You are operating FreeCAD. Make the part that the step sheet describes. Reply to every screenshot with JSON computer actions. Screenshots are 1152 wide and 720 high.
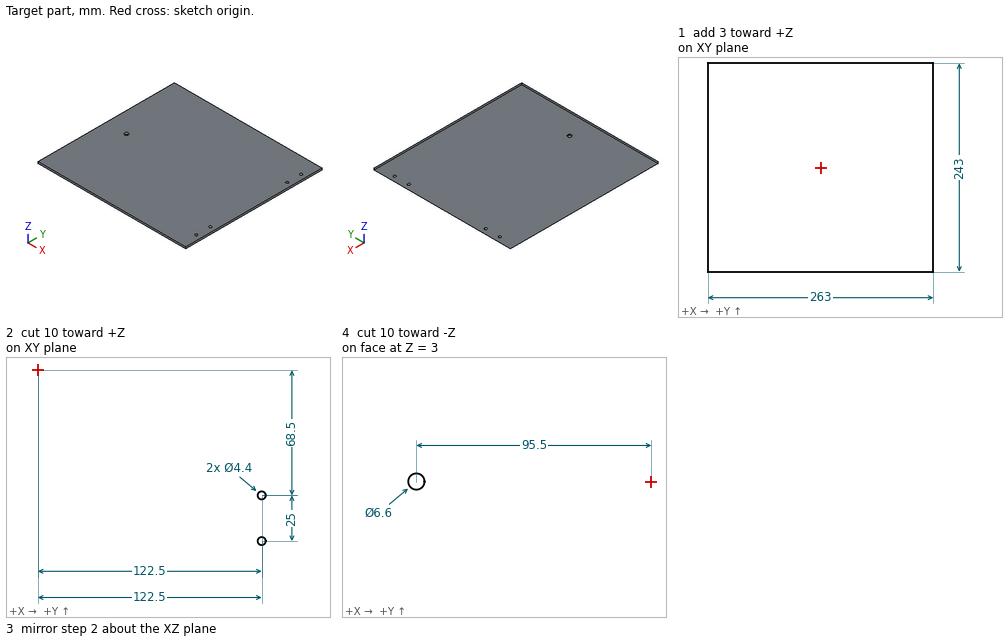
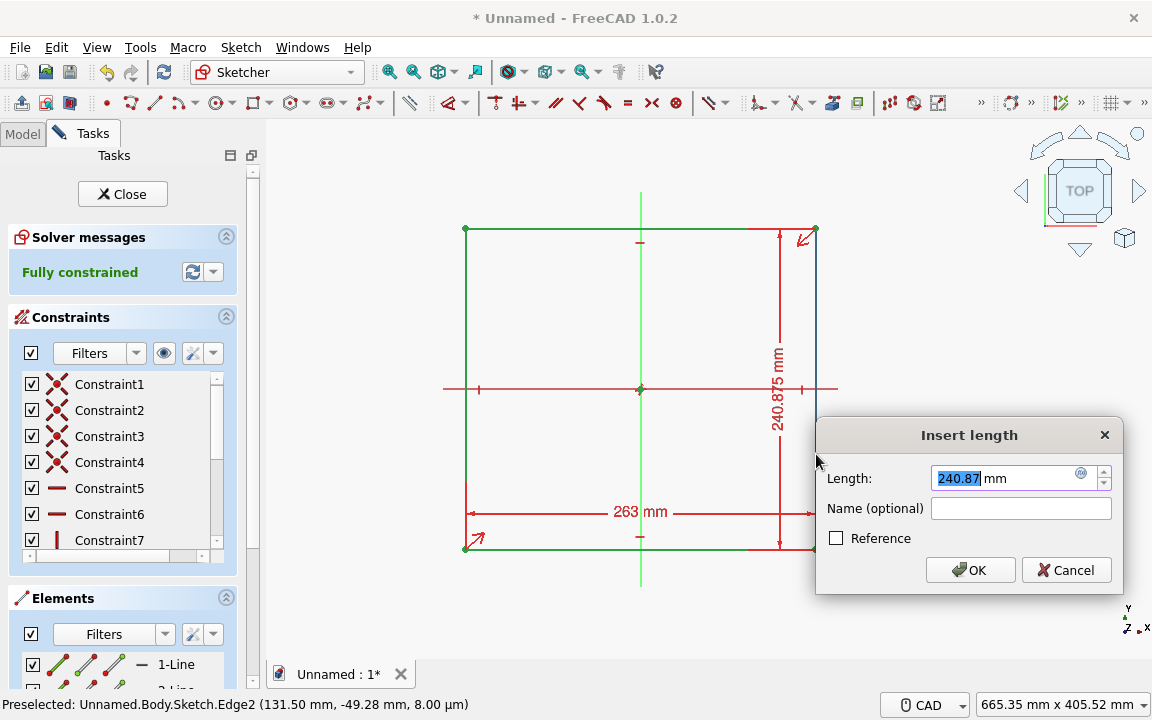
{"action": "type", "text": "243"}
{"action": "key", "text": "Return"}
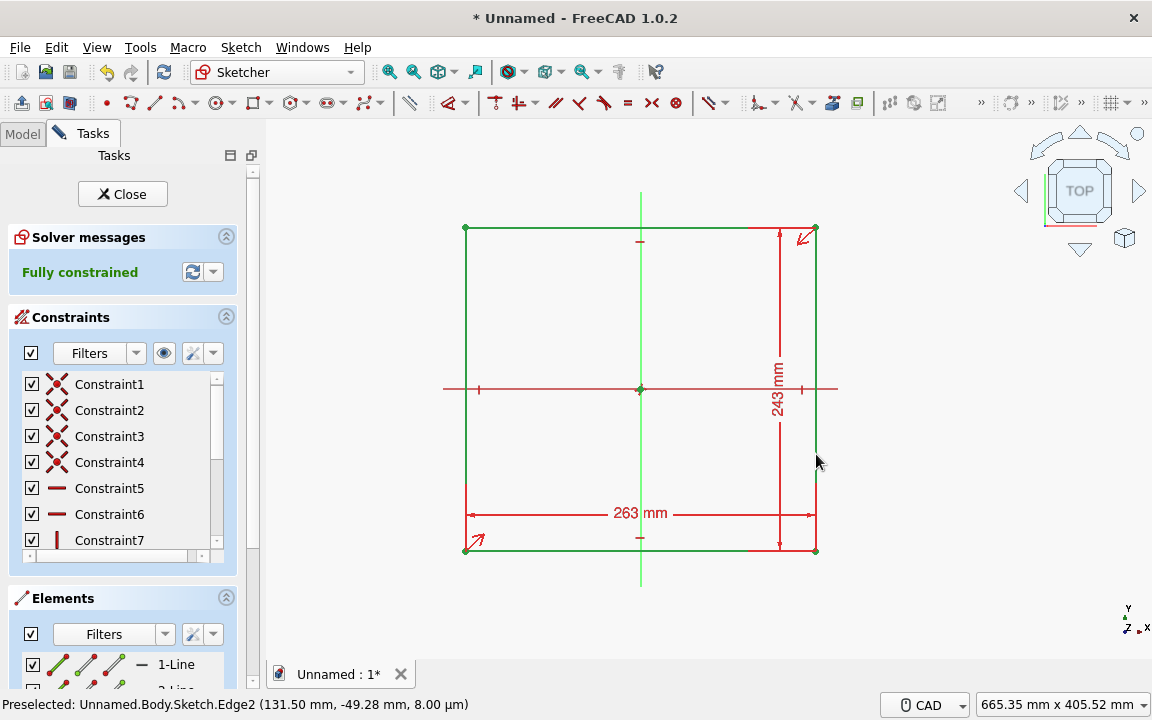
{"action": "left_click", "coordinate": [123, 194]}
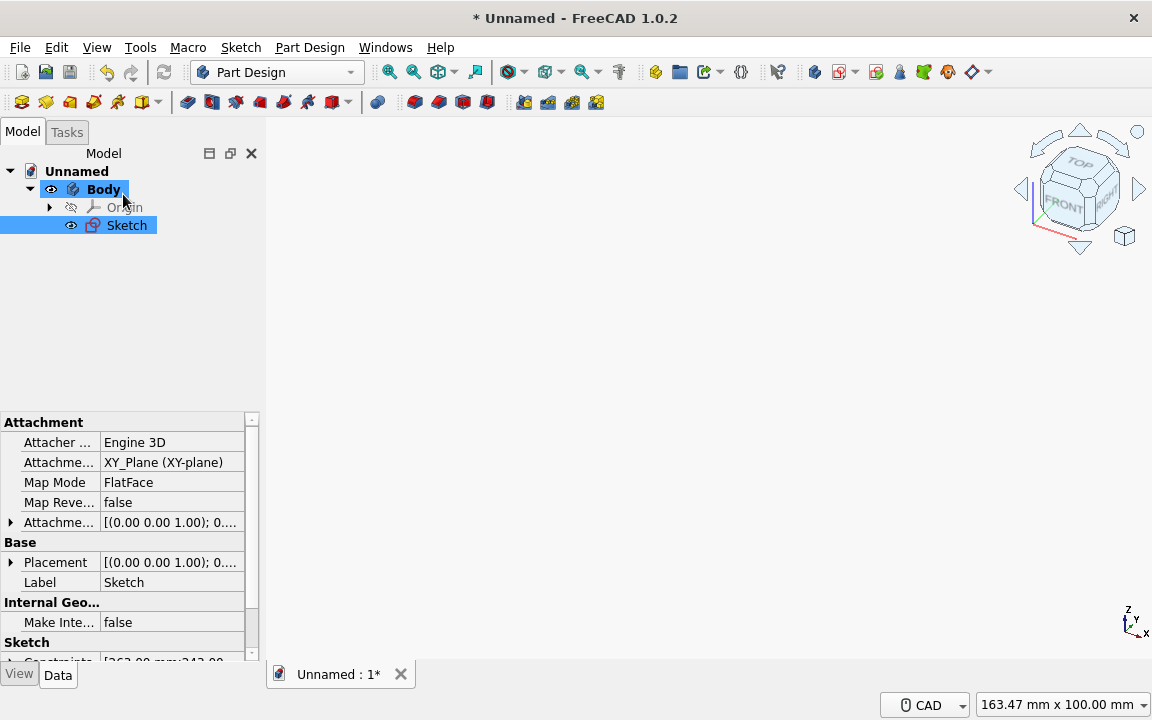
{"action": "left_click", "coordinate": [22, 102]}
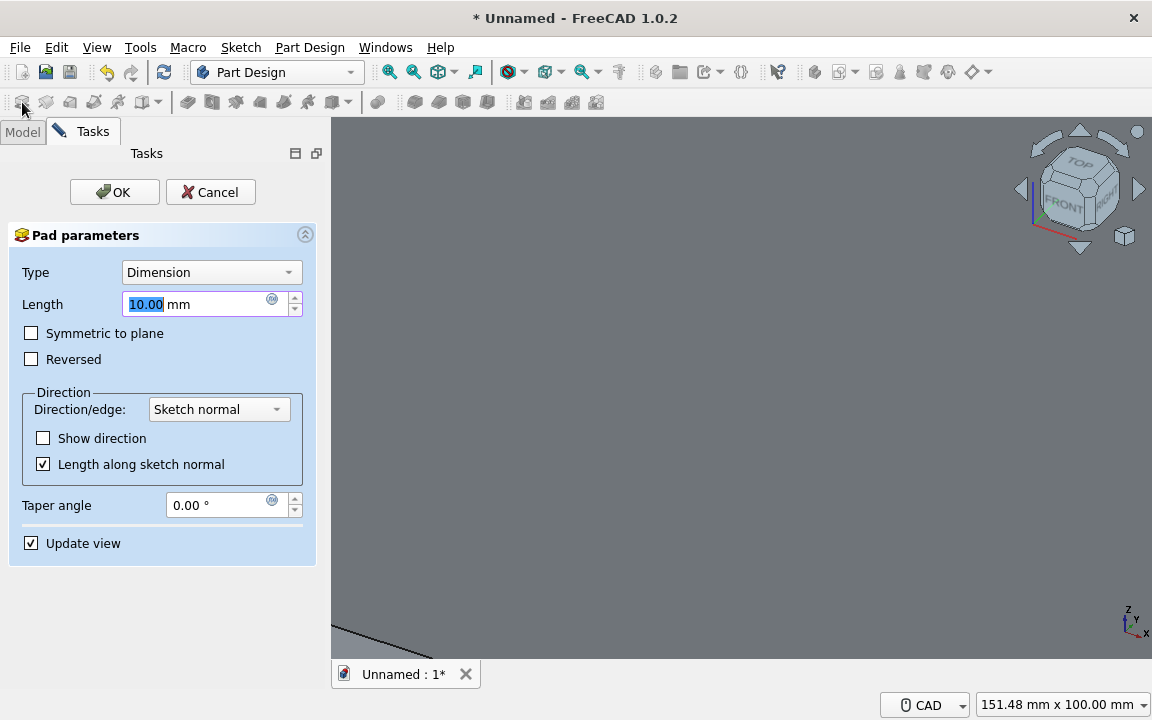
{"action": "type", "text": "3"}
{"action": "key", "text": "Tab"}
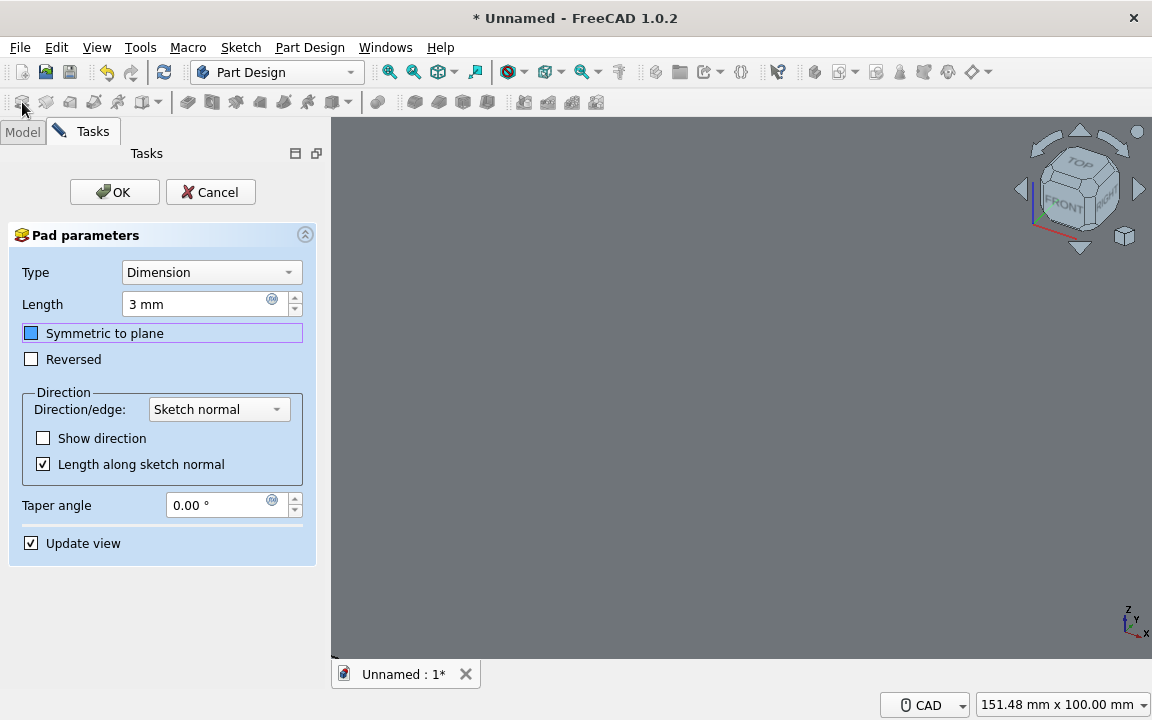
{"action": "left_click", "coordinate": [115, 192]}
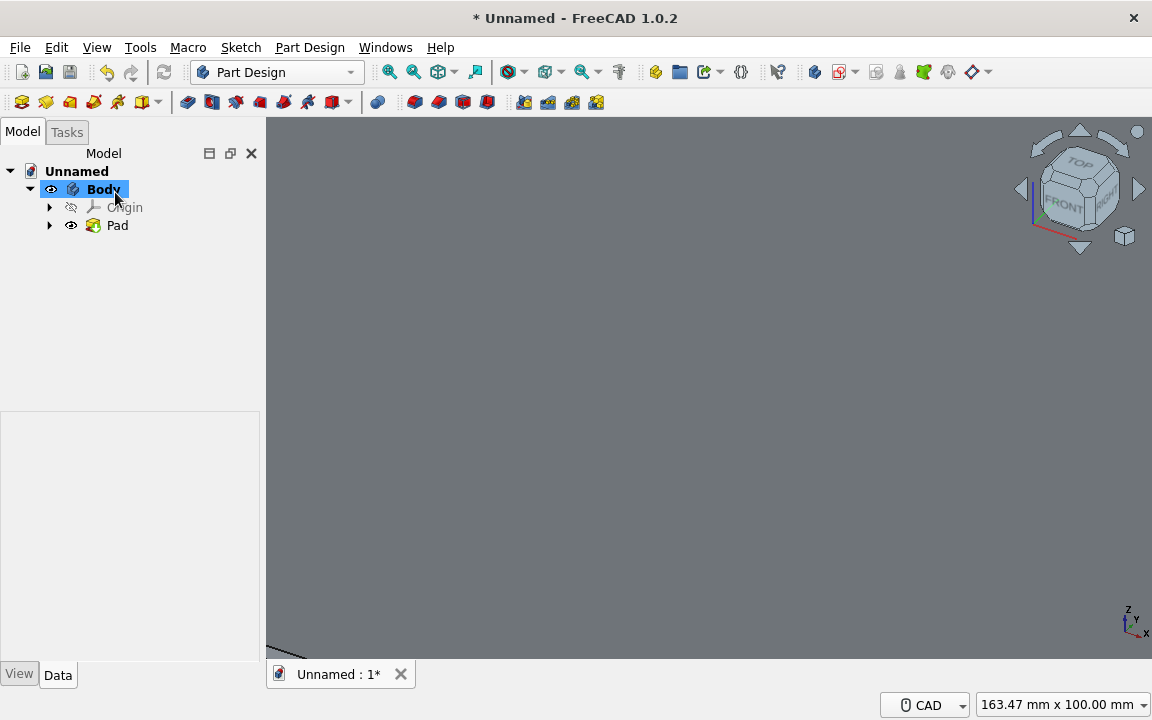
{"action": "key", "text": "v f"}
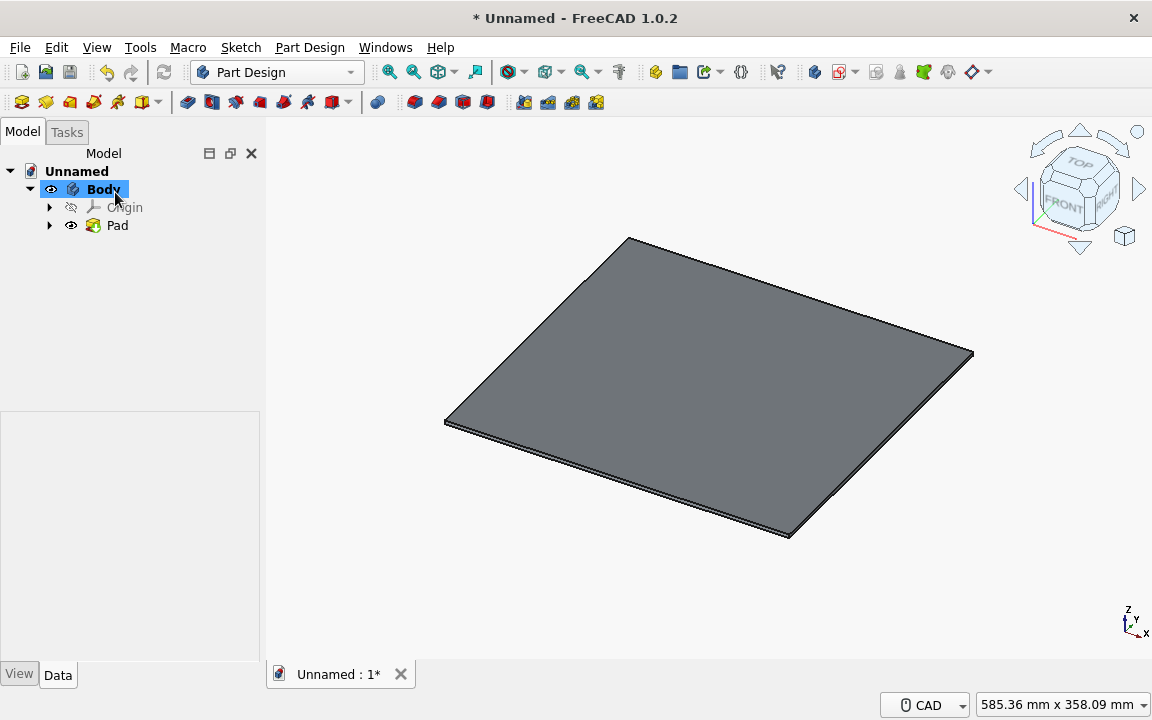
{"action": "left_click", "coordinate": [840, 72]}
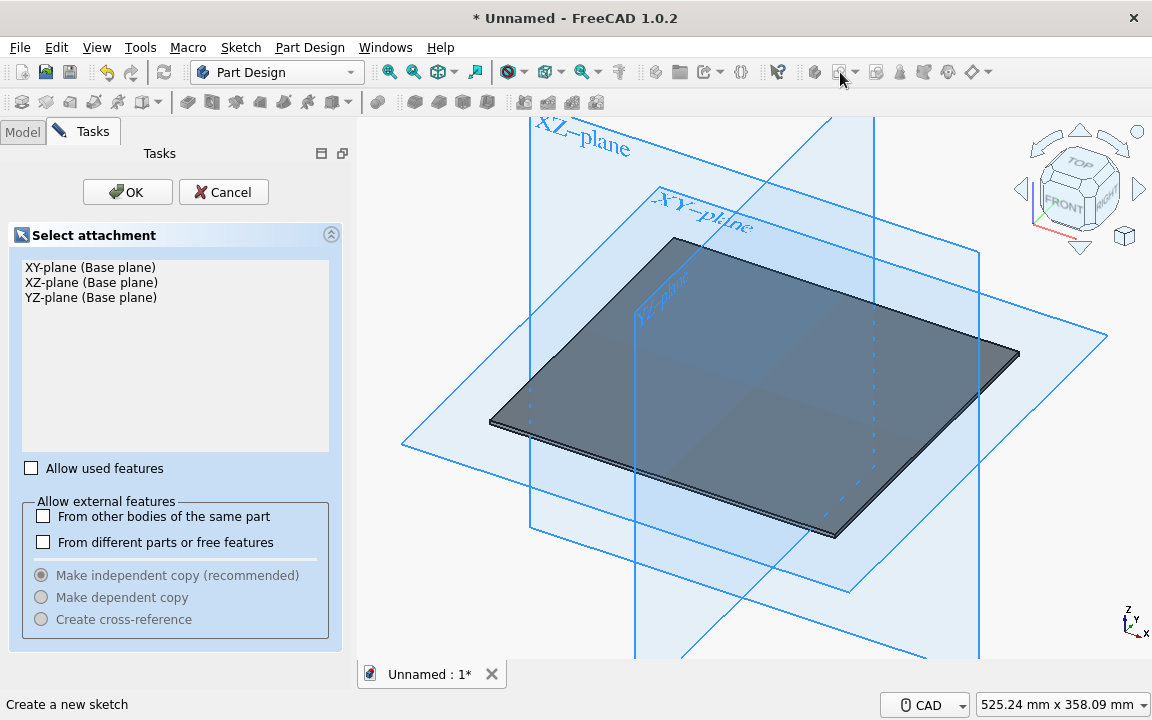
{"action": "left_click", "coordinate": [82, 268]}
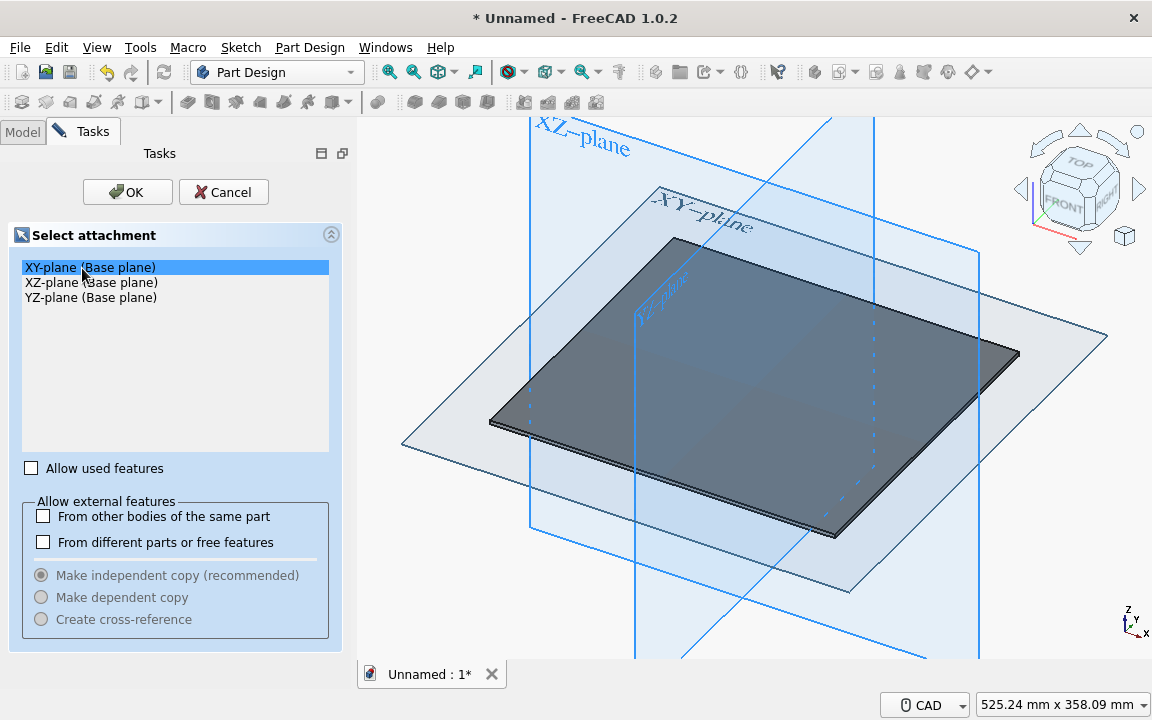
{"action": "left_click", "coordinate": [128, 192]}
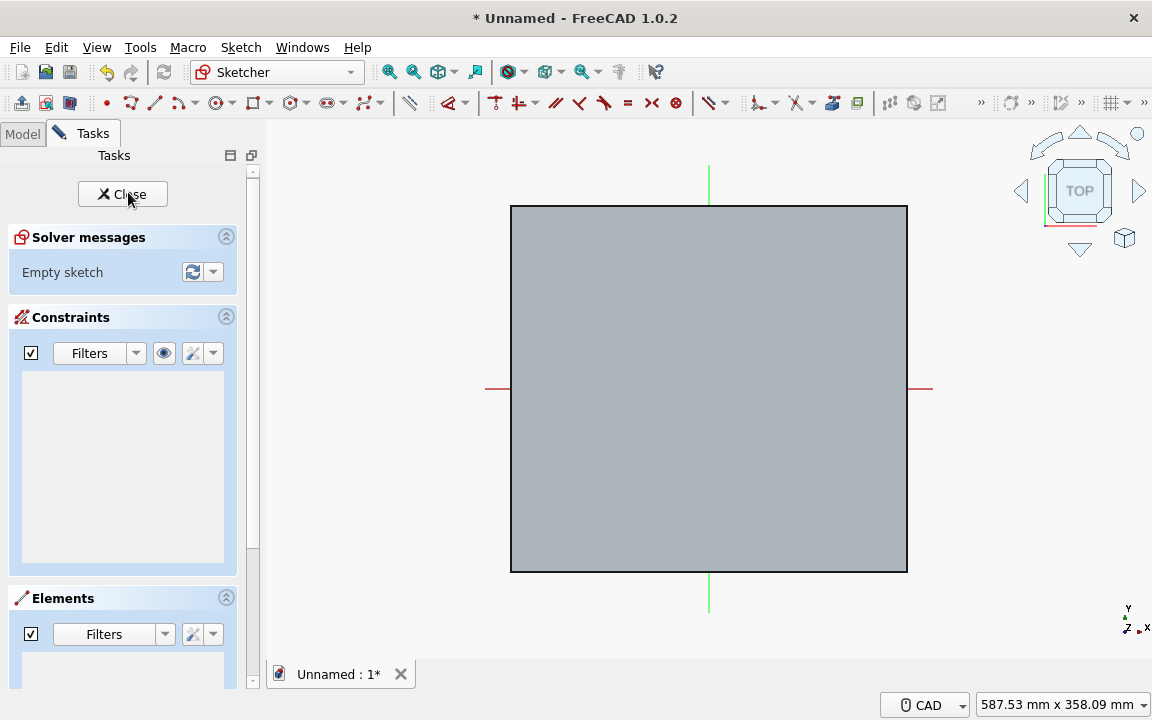
{"action": "key", "text": "q s"}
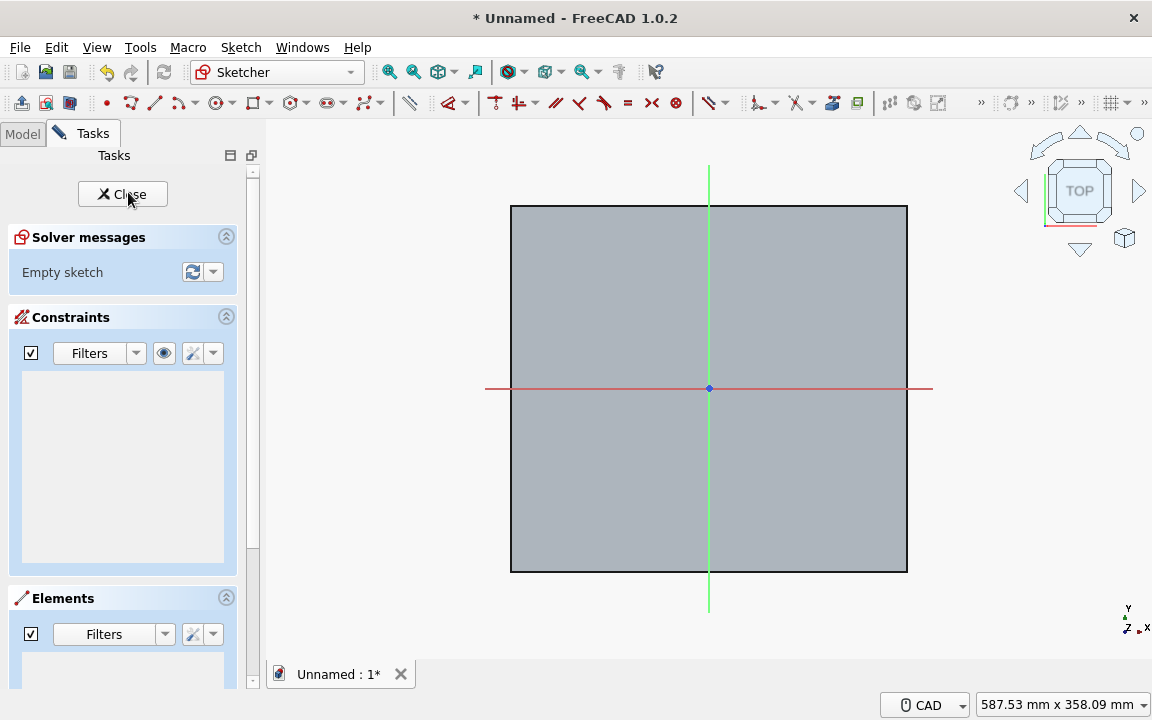
{"action": "scroll", "coordinate": [933, 530], "scroll_direction": "up", "scroll_amount": 10}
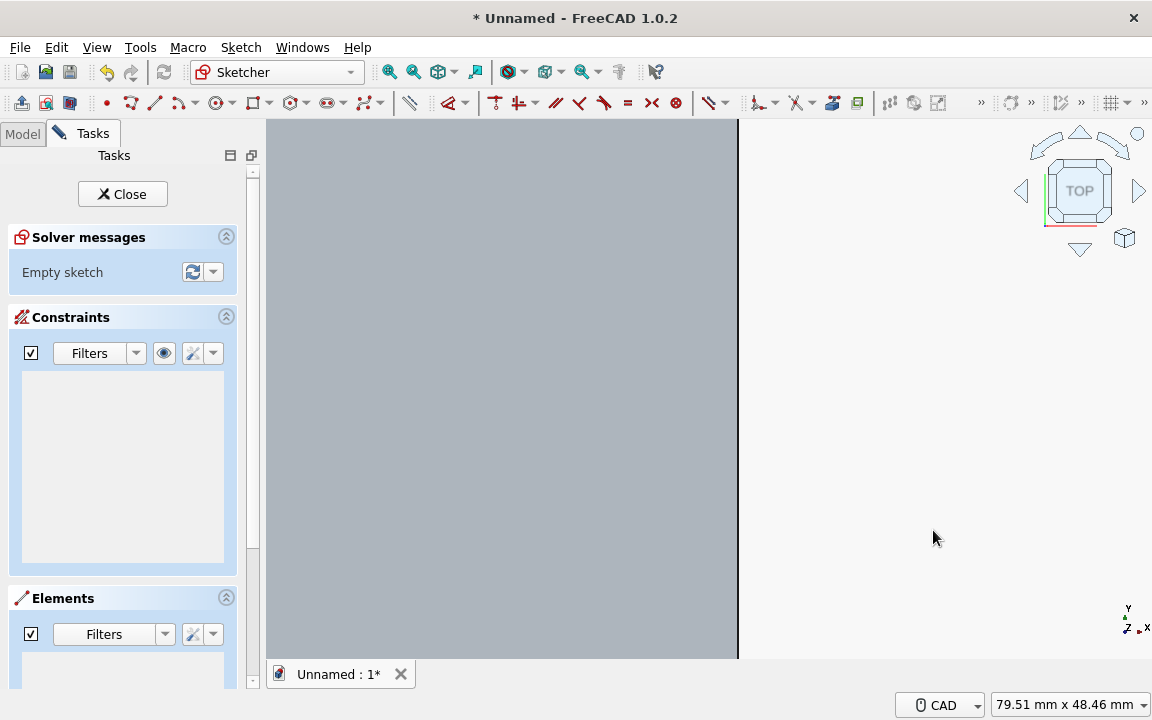
{"action": "left_click", "coordinate": [216, 104]}